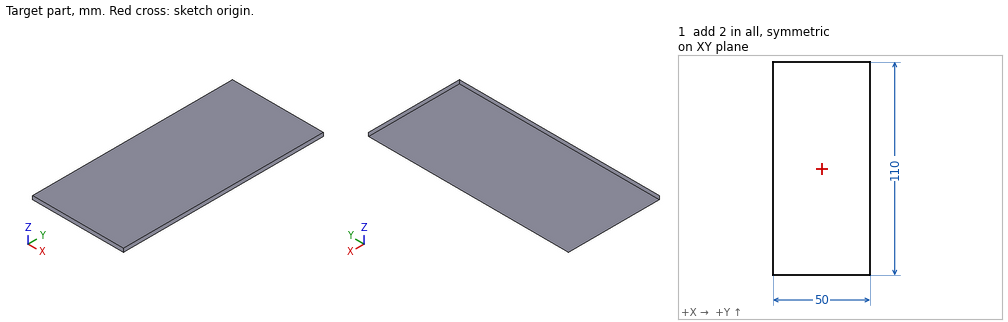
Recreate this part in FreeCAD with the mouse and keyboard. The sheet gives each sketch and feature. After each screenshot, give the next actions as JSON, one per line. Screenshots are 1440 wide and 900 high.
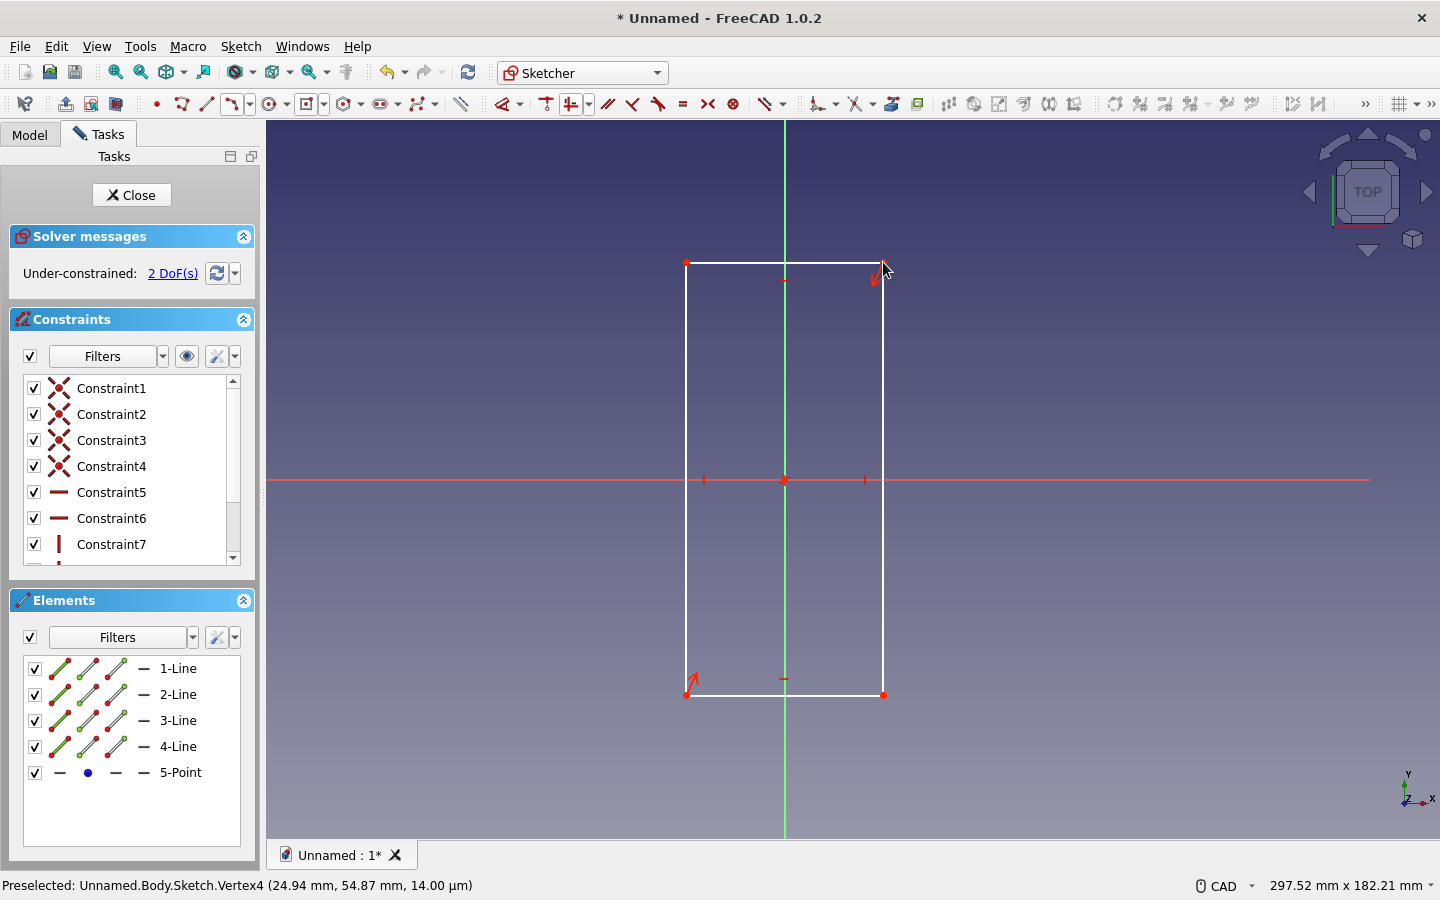
{"action": "left_click", "coordinate": [745, 696]}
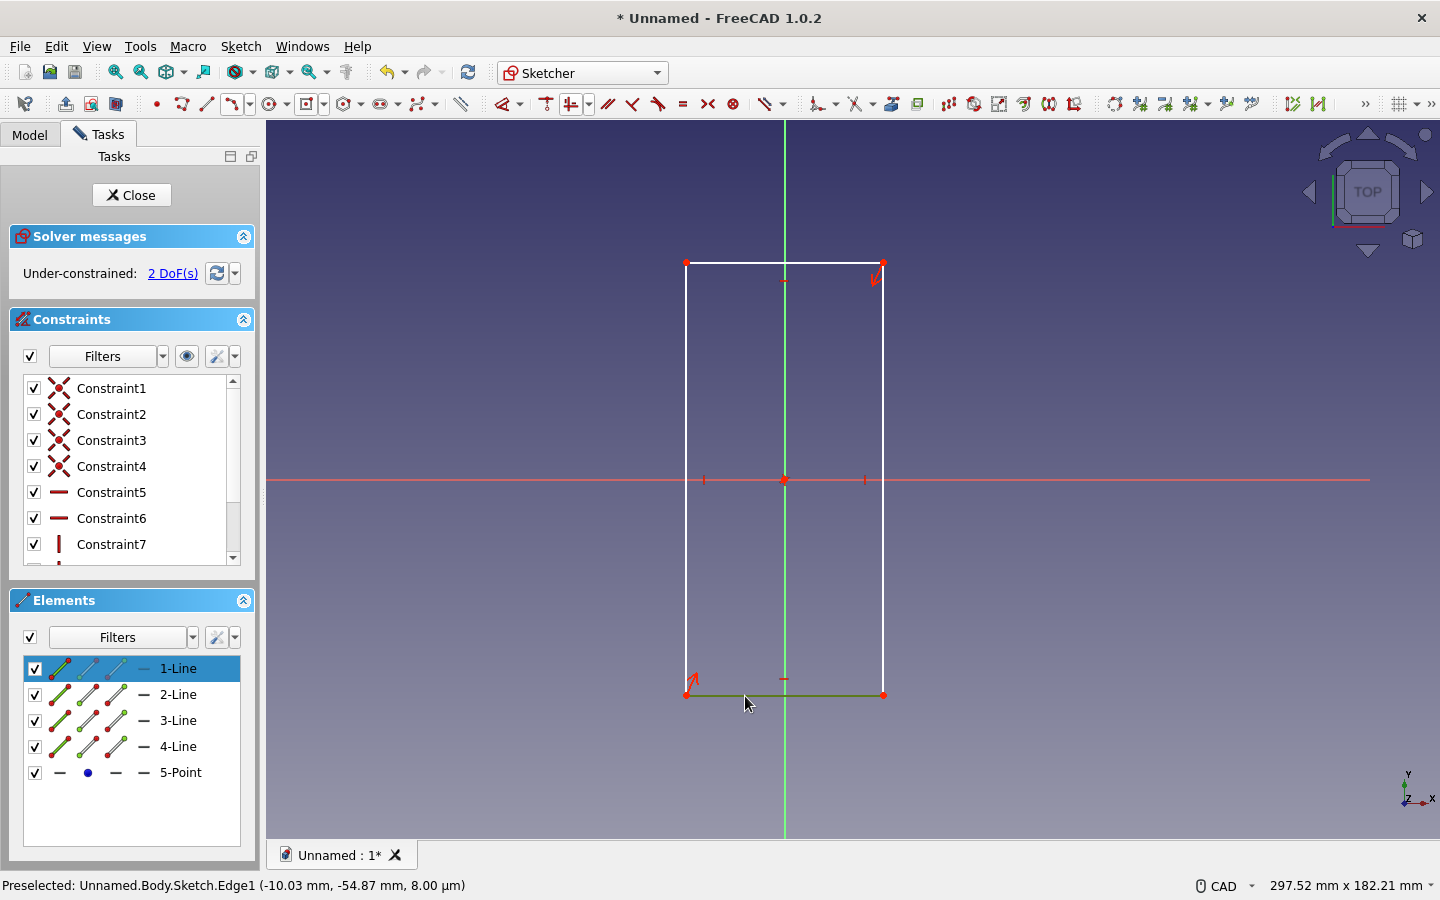
{"action": "key", "text": "l"}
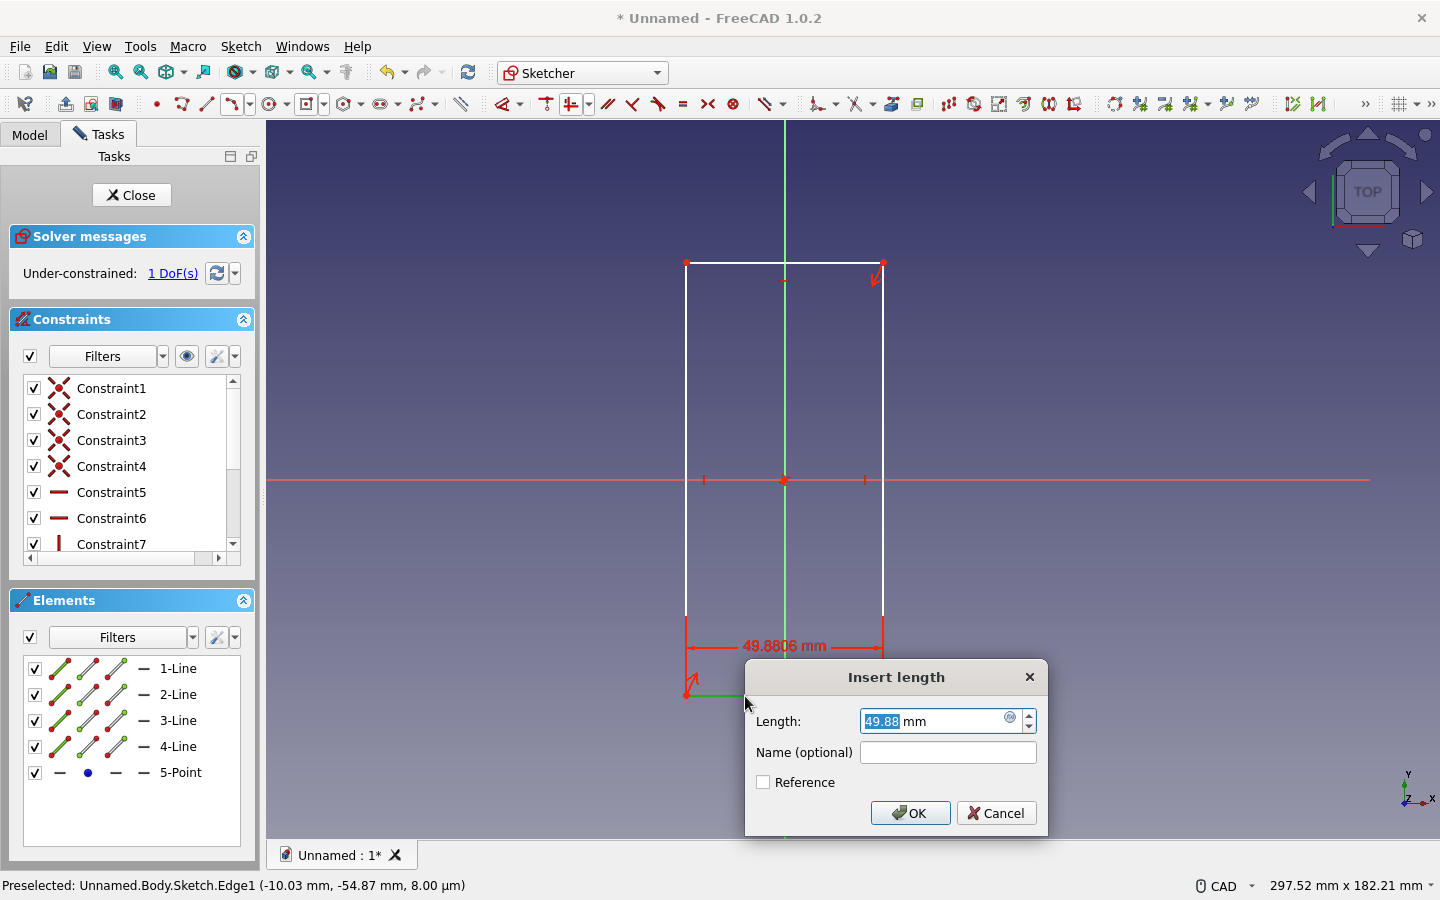
{"action": "type", "text": "50"}
{"action": "key", "text": "Return"}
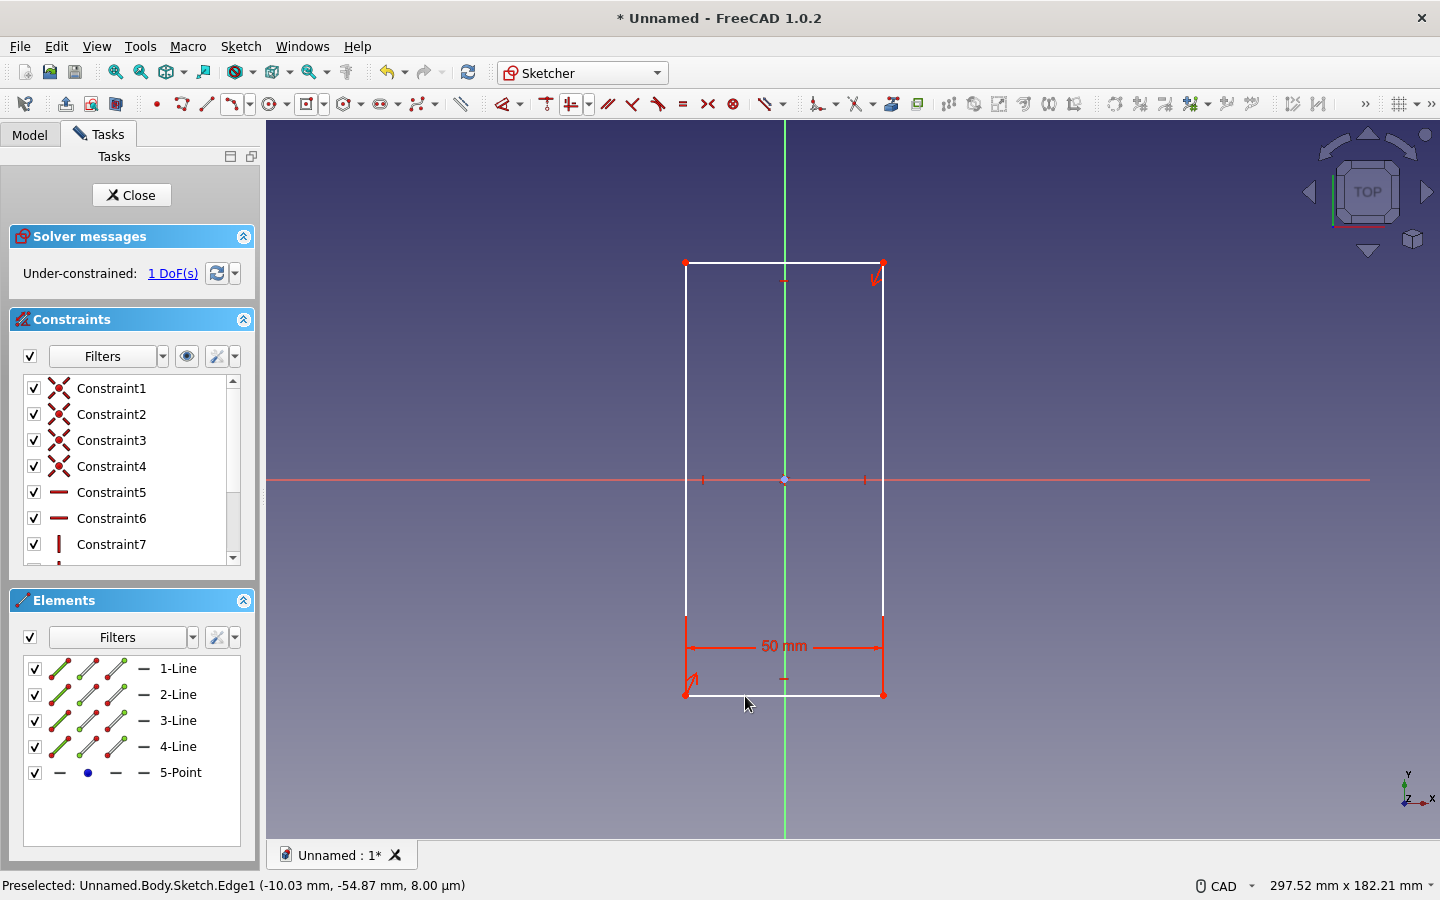
{"action": "left_click", "coordinate": [883, 566]}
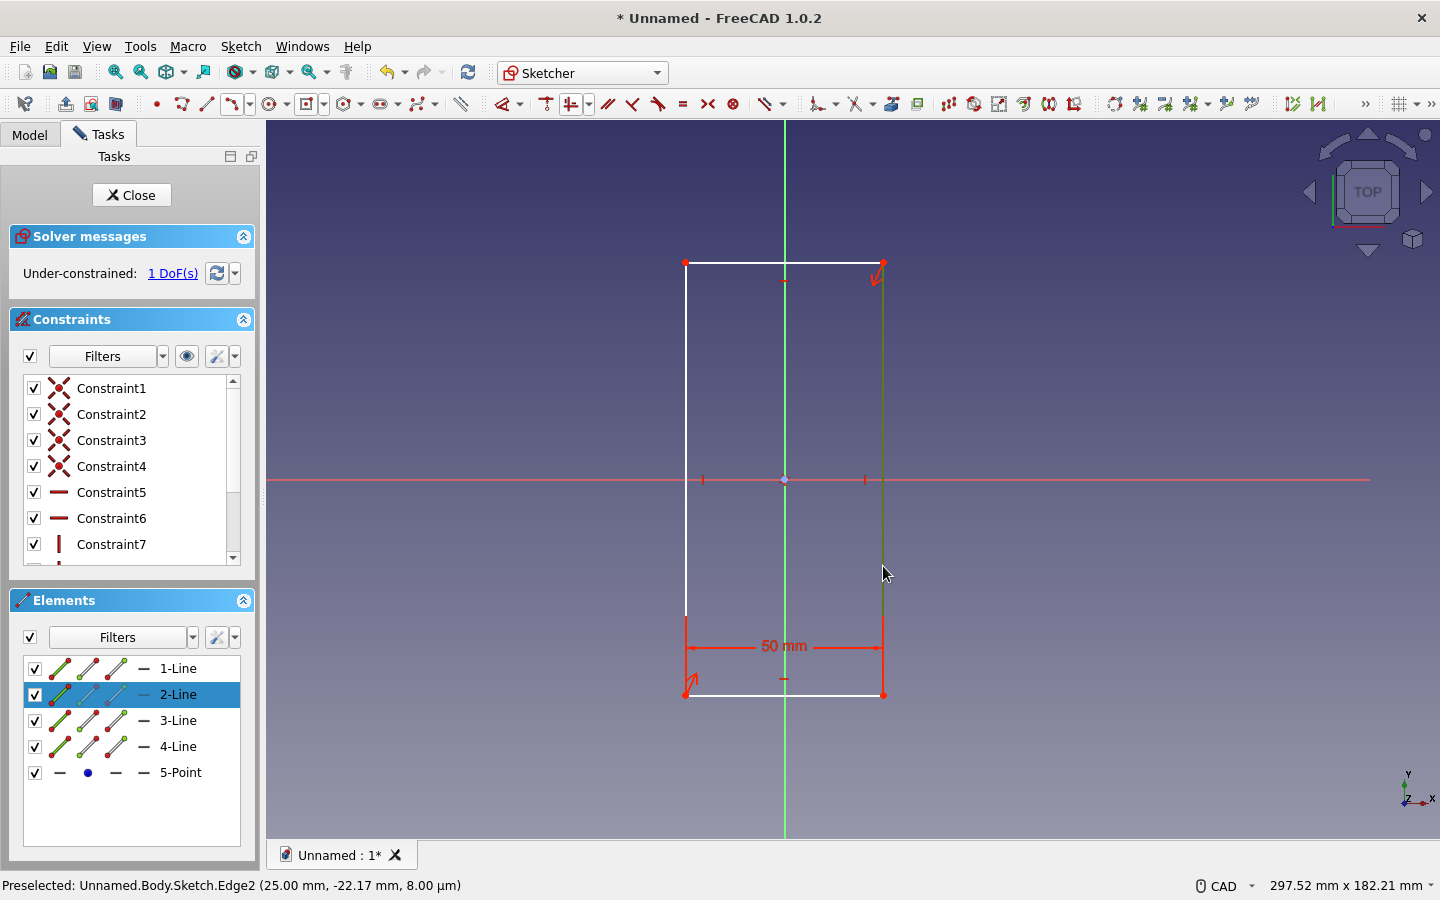
{"action": "key", "text": "i"}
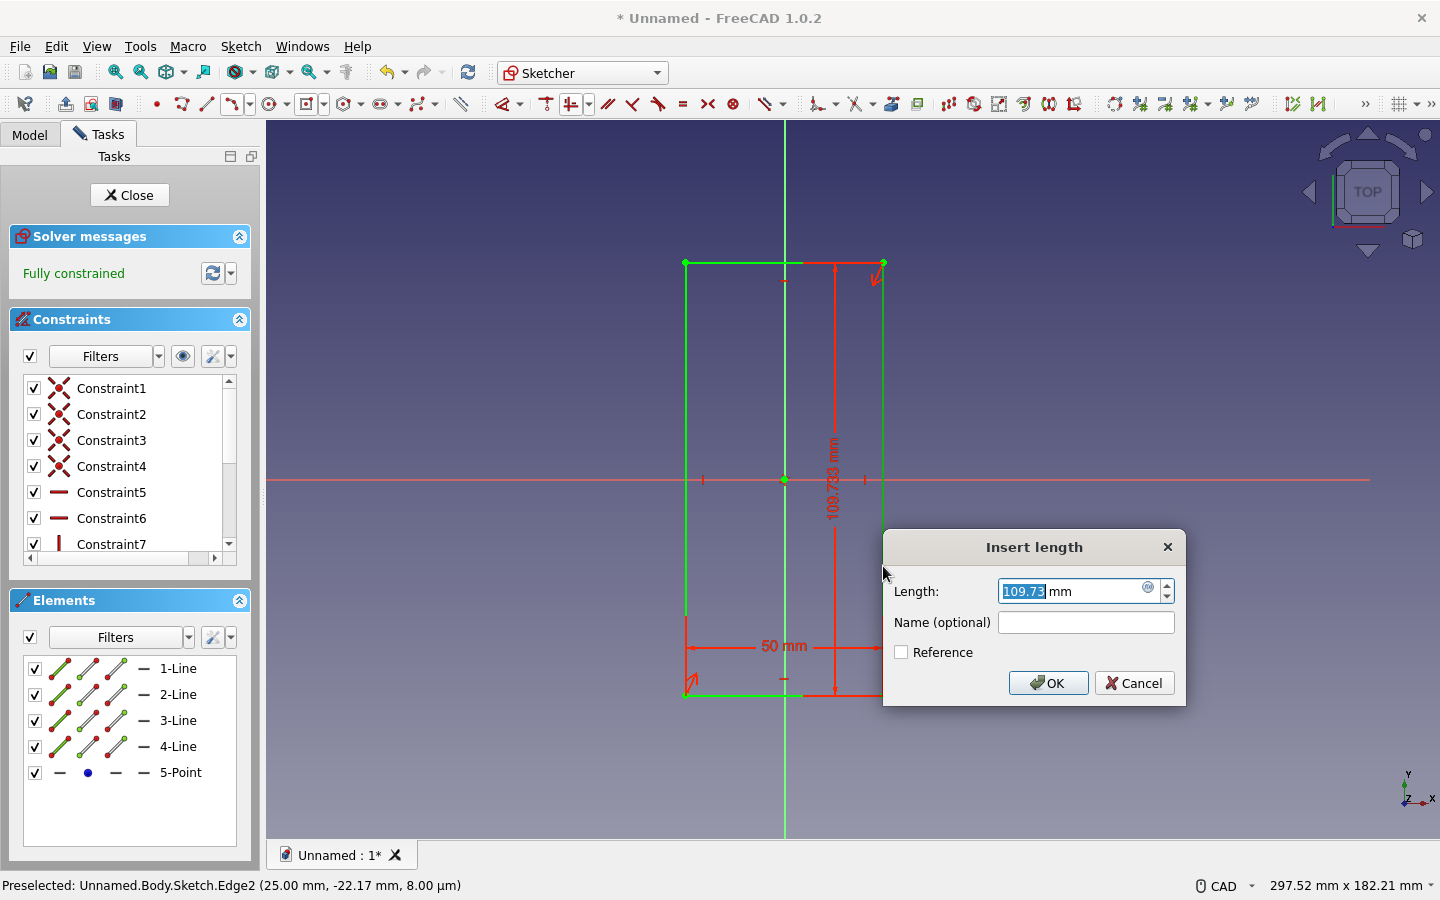
{"action": "type", "text": "110"}
{"action": "key", "text": "Return"}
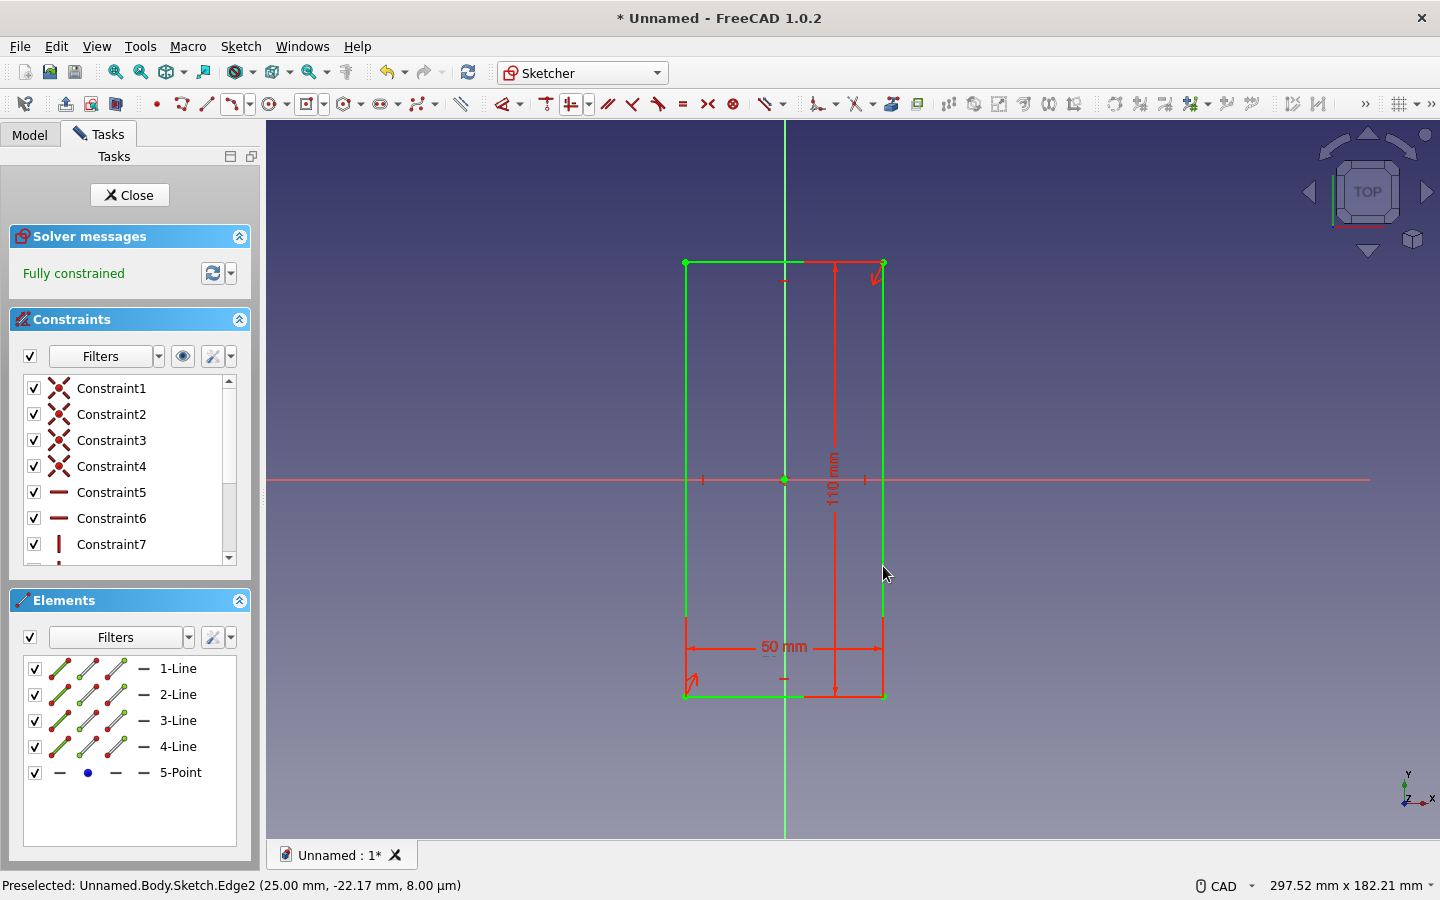
{"action": "left_click", "coordinate": [130, 195]}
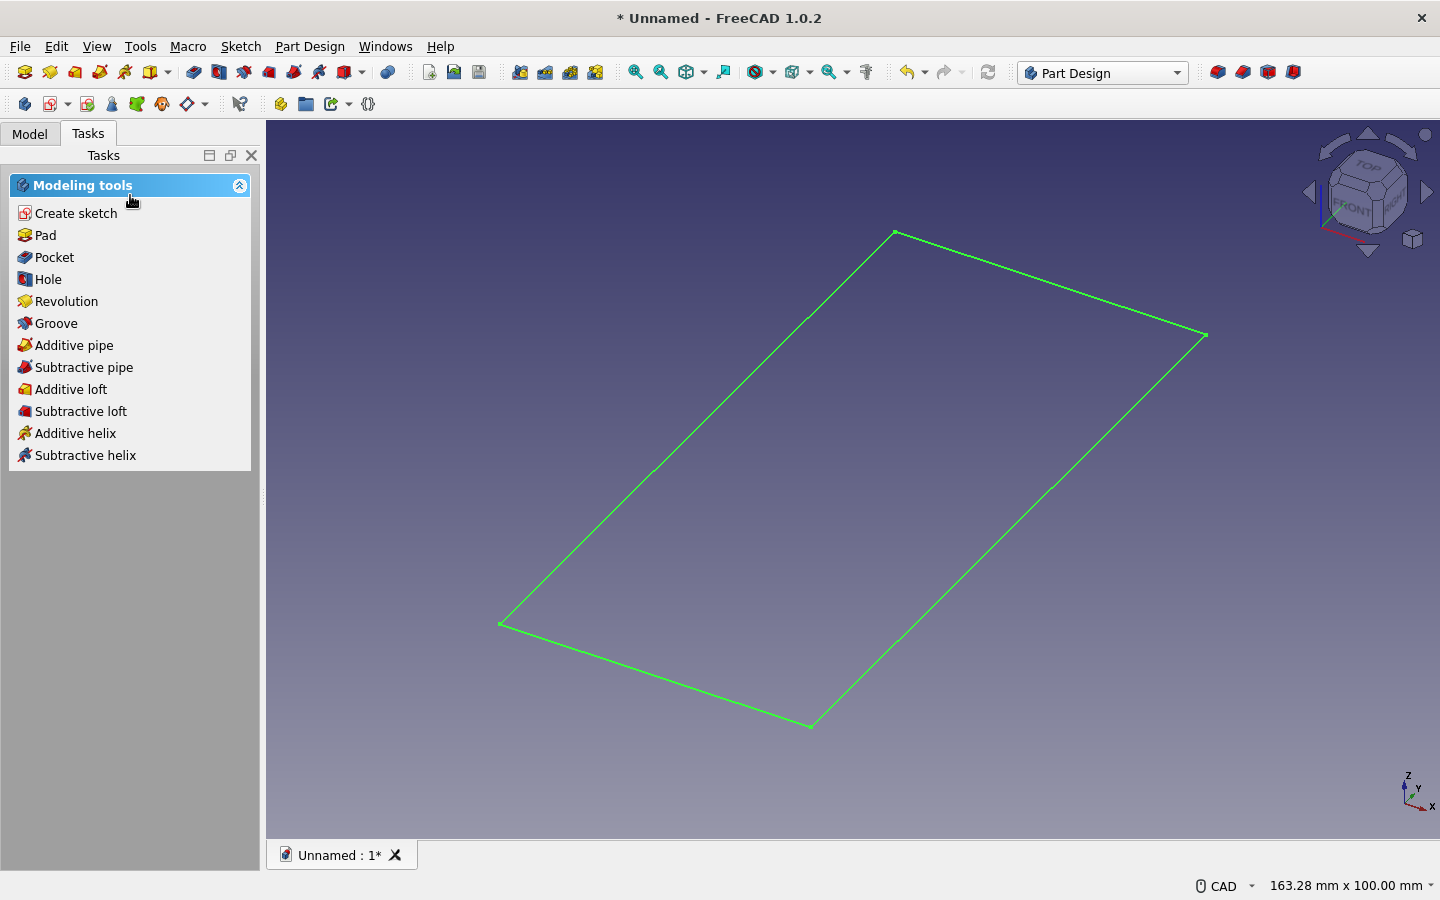
{"action": "left_click", "coordinate": [25, 72]}